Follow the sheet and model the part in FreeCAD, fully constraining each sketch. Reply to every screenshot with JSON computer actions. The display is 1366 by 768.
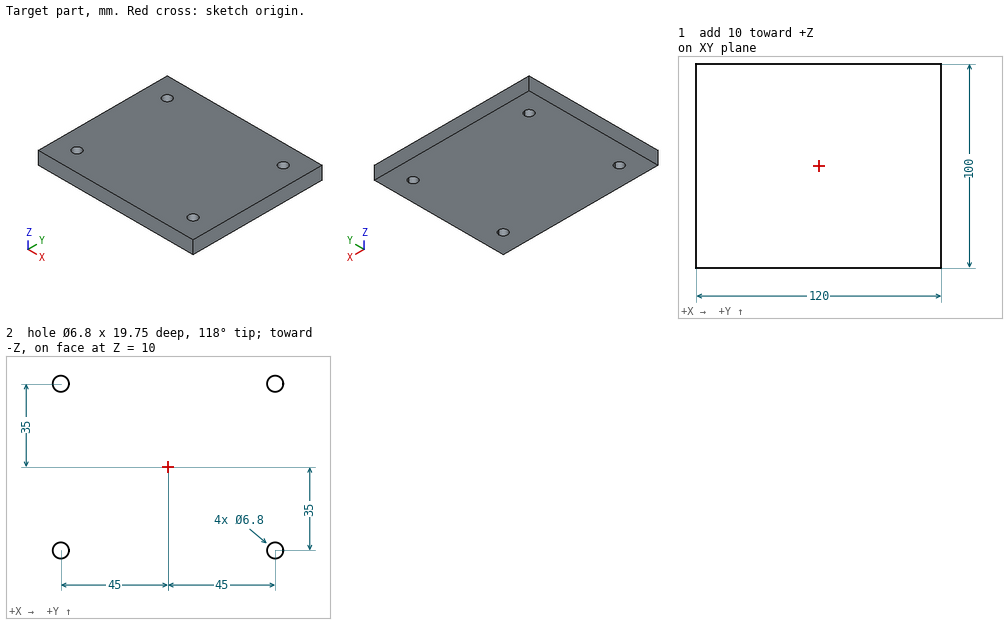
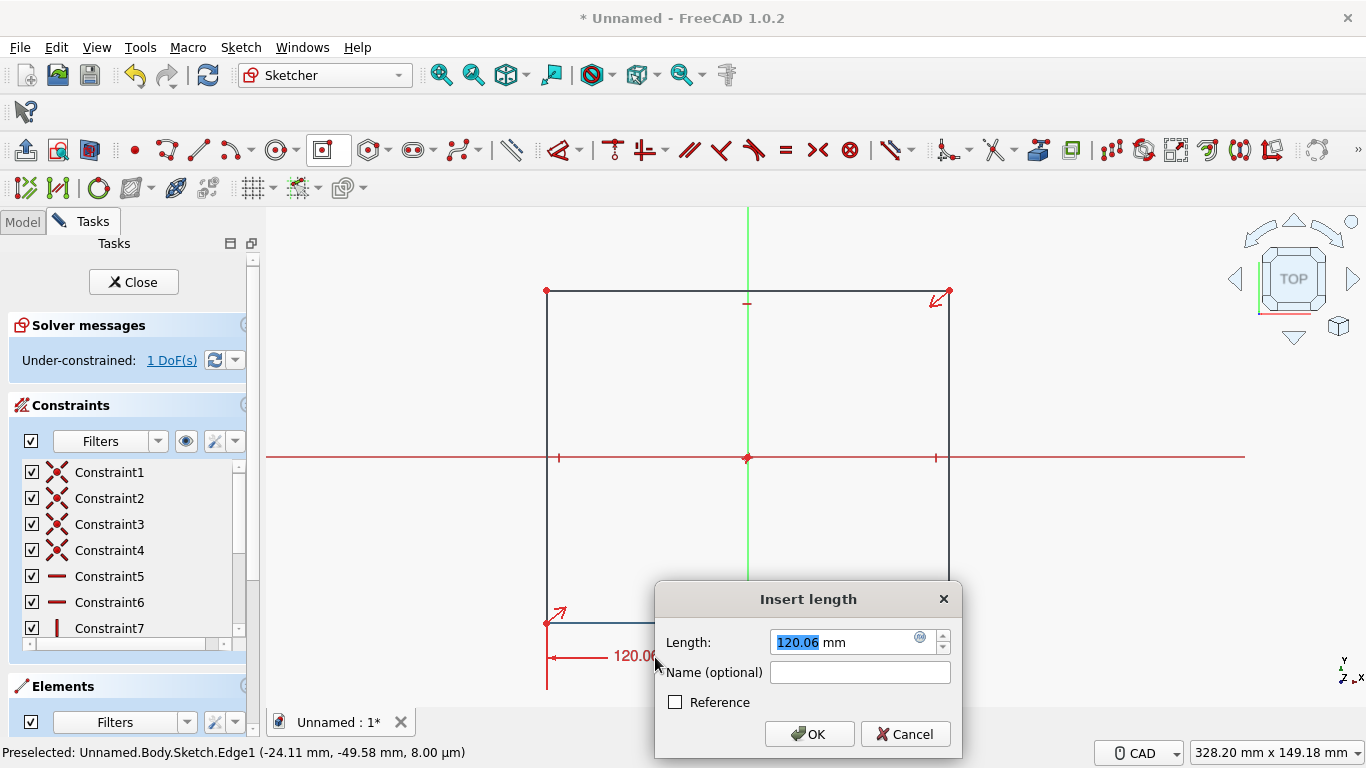
{"action": "type", "text": "120"}
{"action": "key", "text": "Return"}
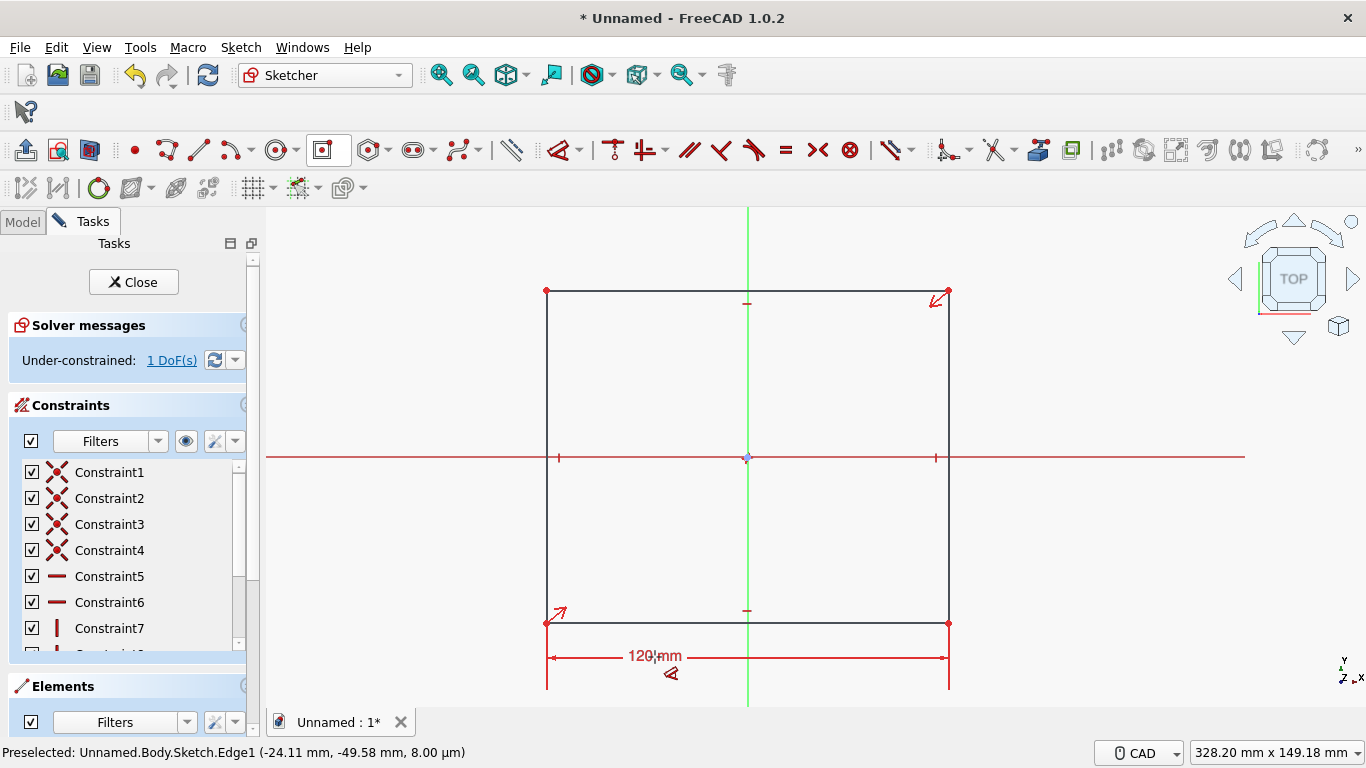
{"action": "left_click", "coordinate": [949, 524]}
{"action": "left_click", "coordinate": [983, 381]}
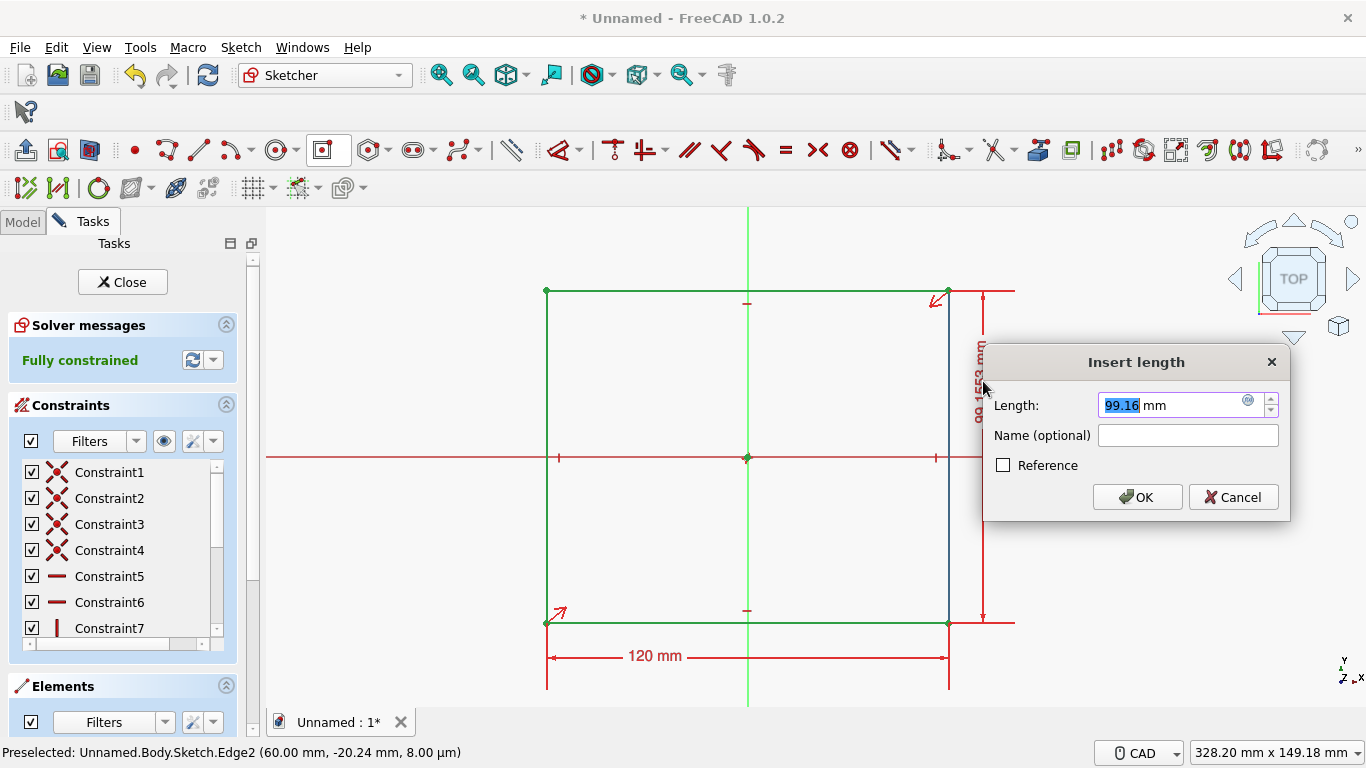
{"action": "type", "text": "100"}
{"action": "key", "text": "Return"}
{"action": "key", "text": "Escape"}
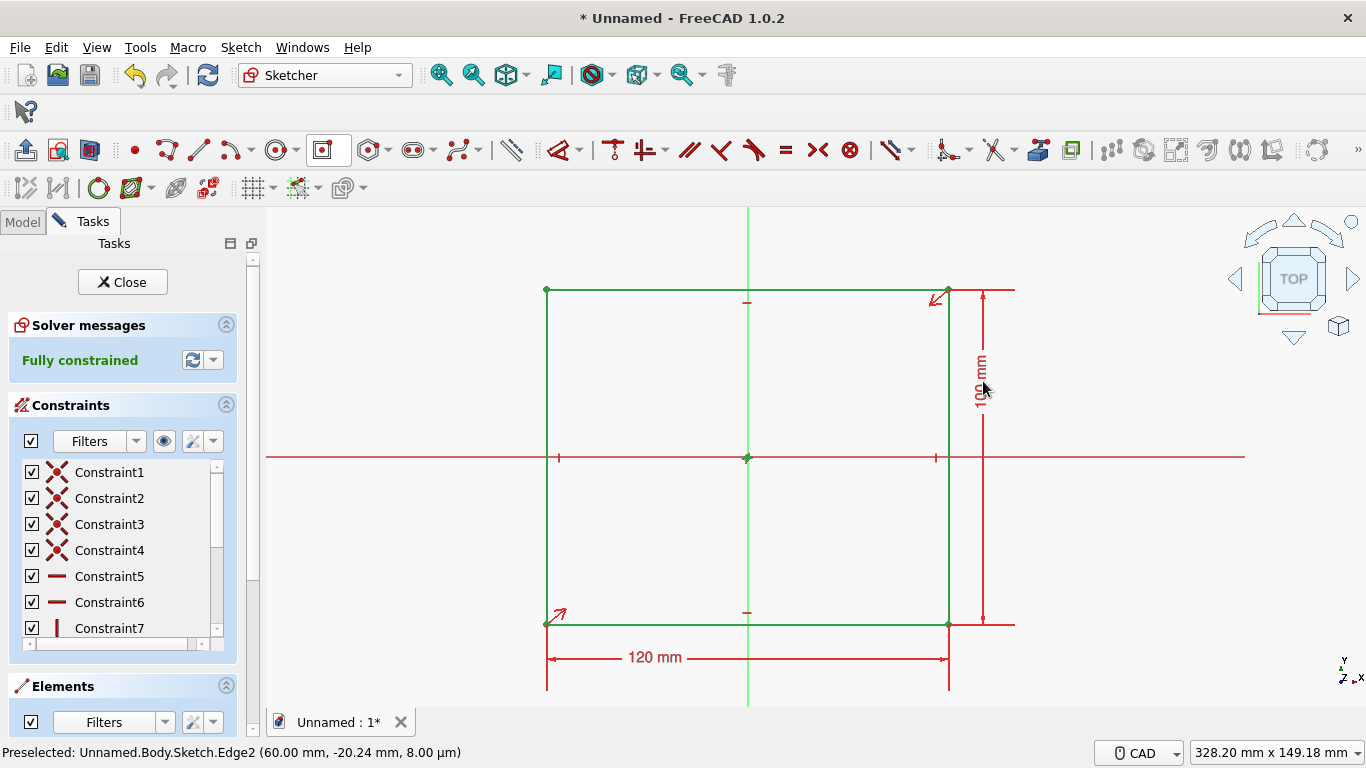
{"action": "left_click", "coordinate": [123, 282]}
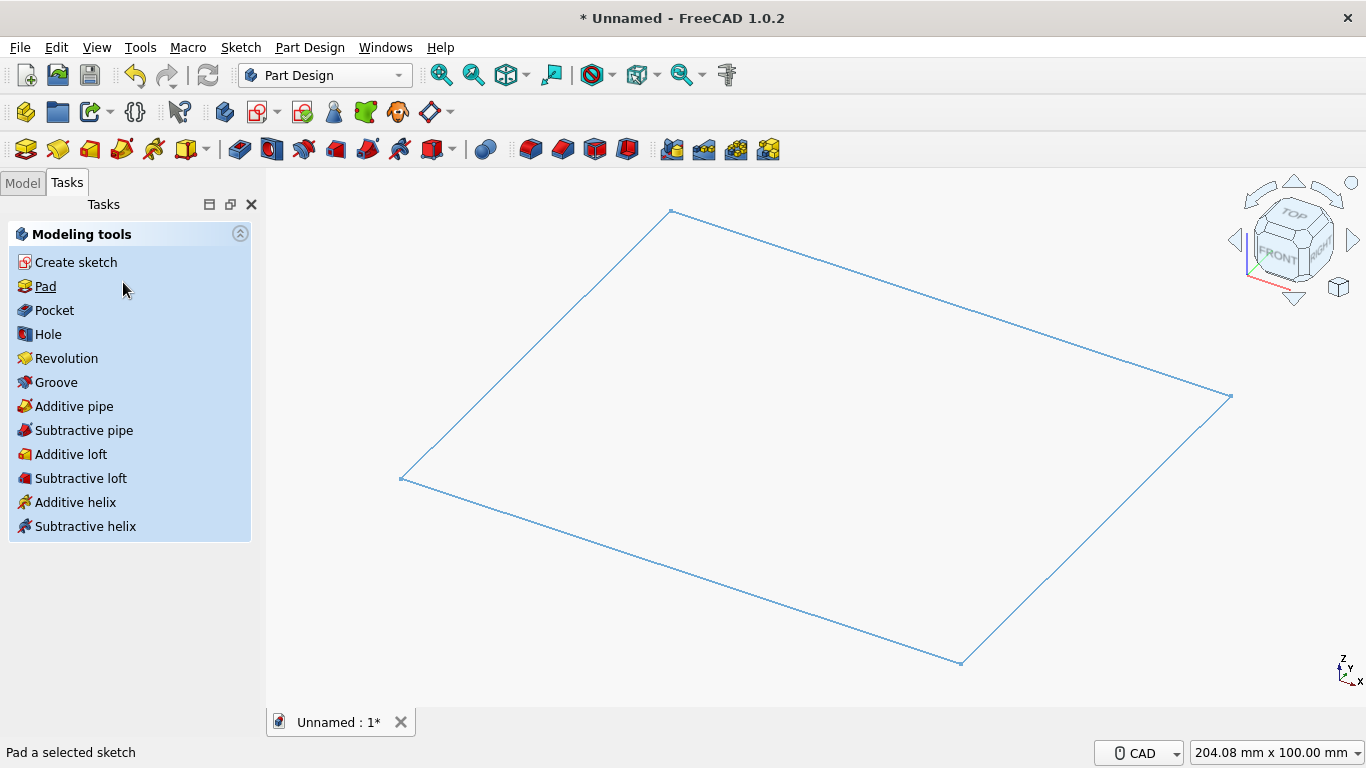
{"action": "left_click", "coordinate": [26, 150]}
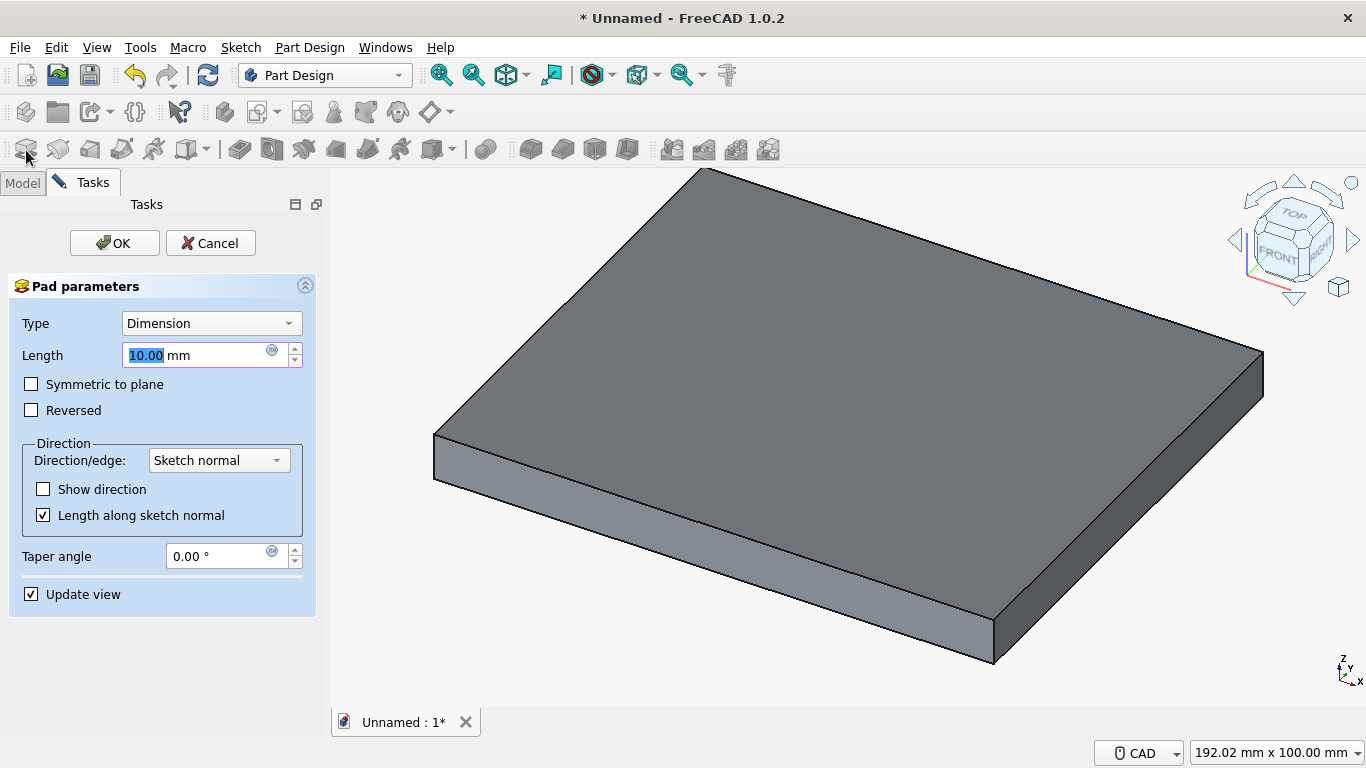
{"action": "type", "text": "10"}
{"action": "key", "text": "Tab"}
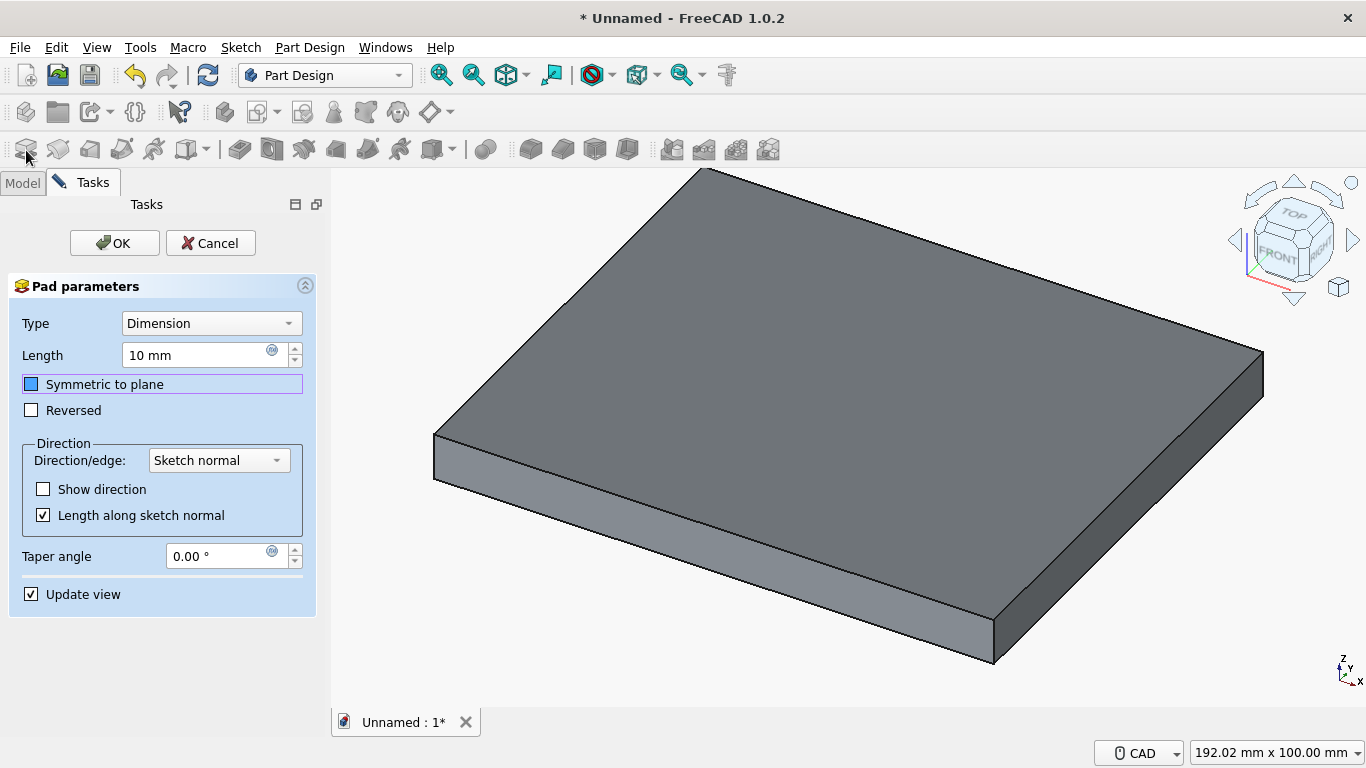
{"action": "left_click", "coordinate": [115, 243]}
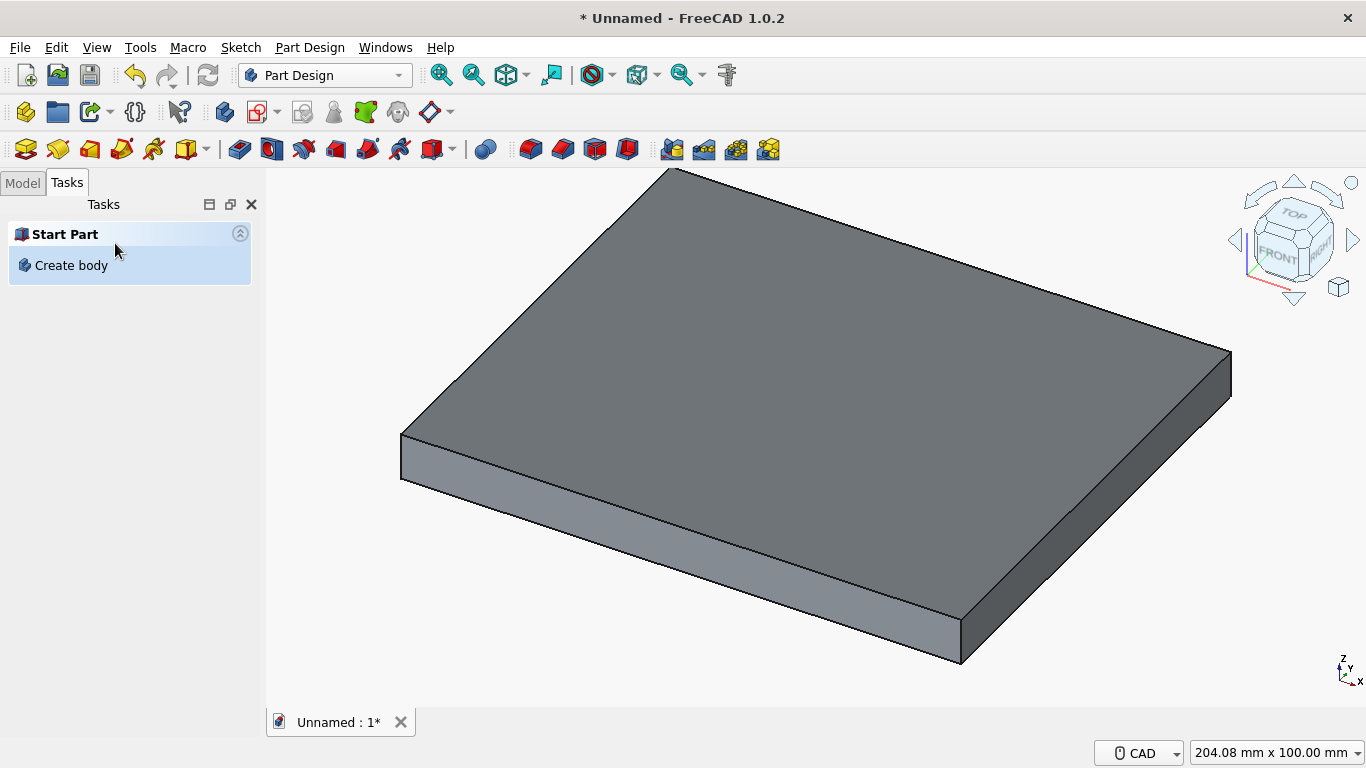
{"action": "left_click", "coordinate": [442, 76]}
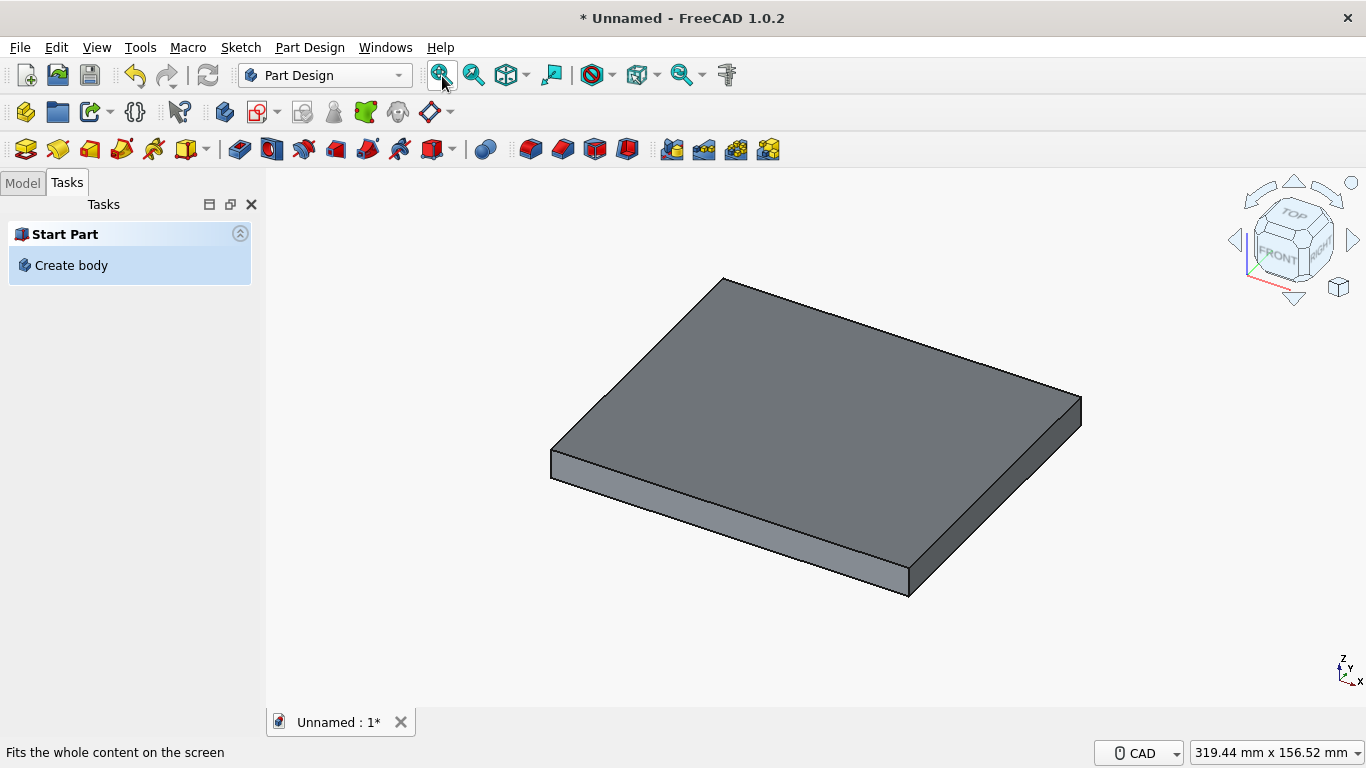
{"action": "left_click", "coordinate": [816, 422]}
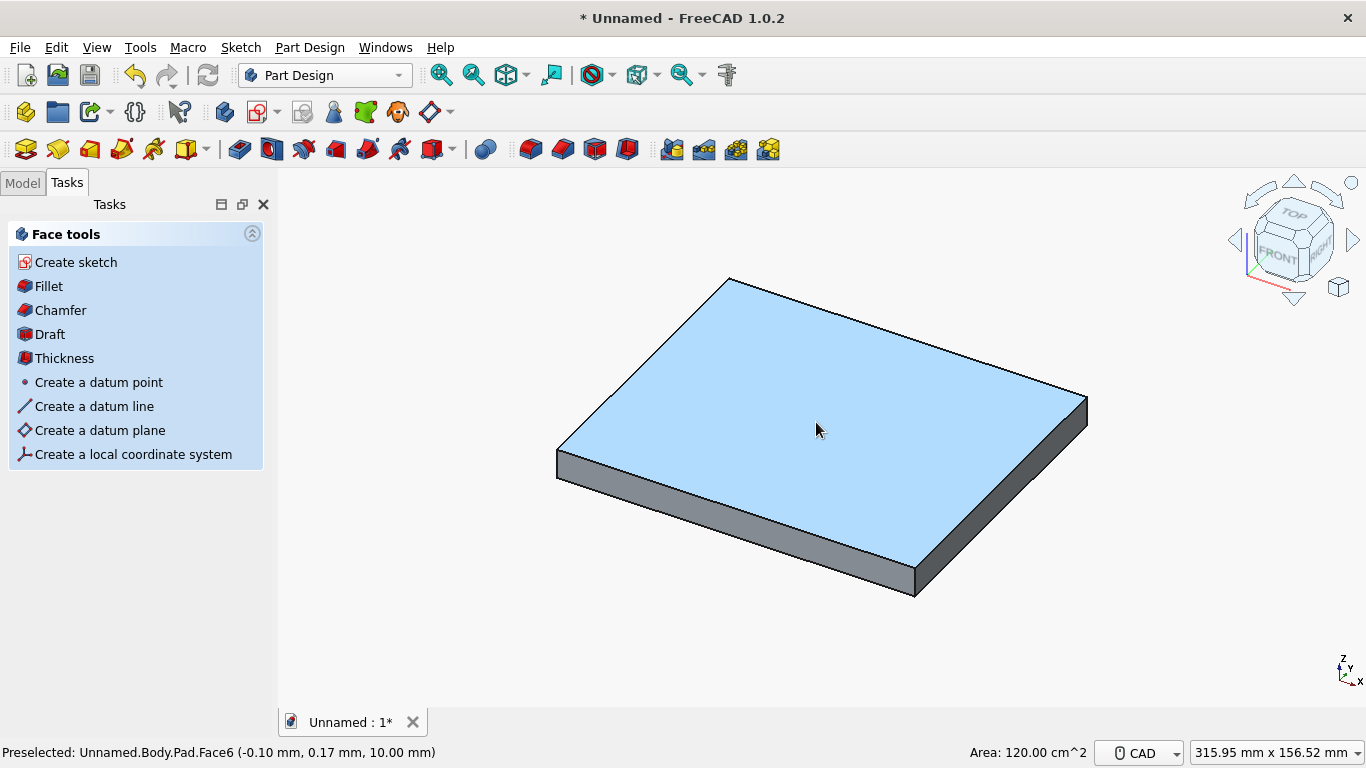
{"action": "left_click", "coordinate": [258, 112]}